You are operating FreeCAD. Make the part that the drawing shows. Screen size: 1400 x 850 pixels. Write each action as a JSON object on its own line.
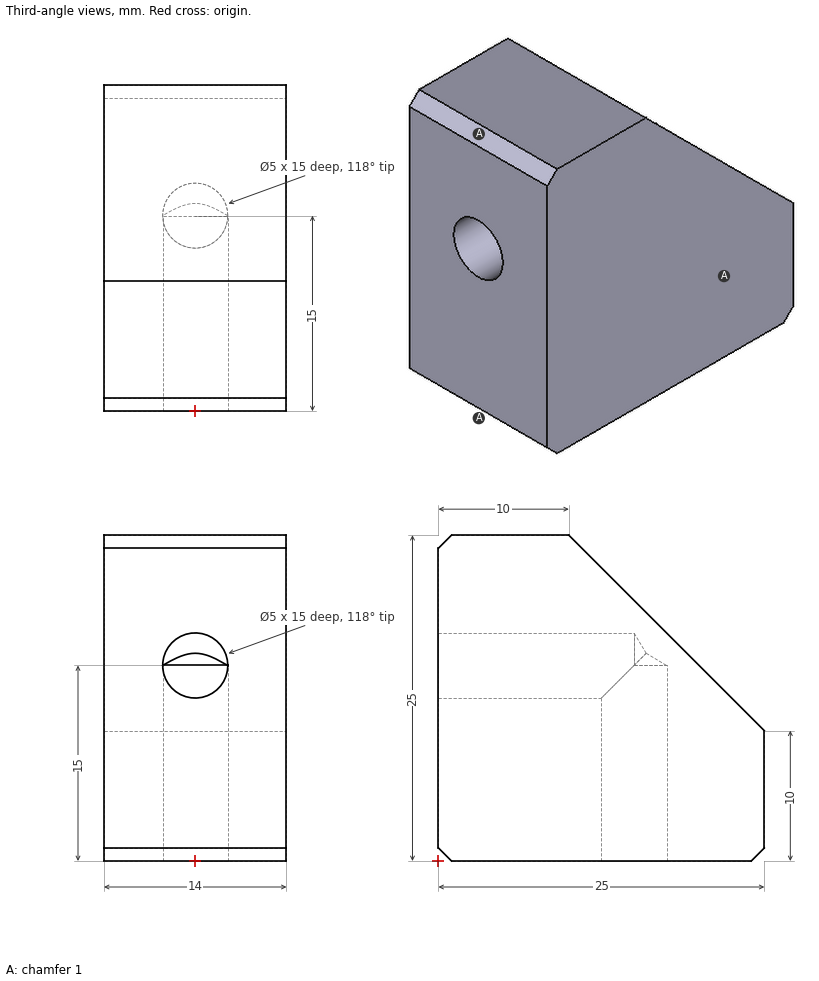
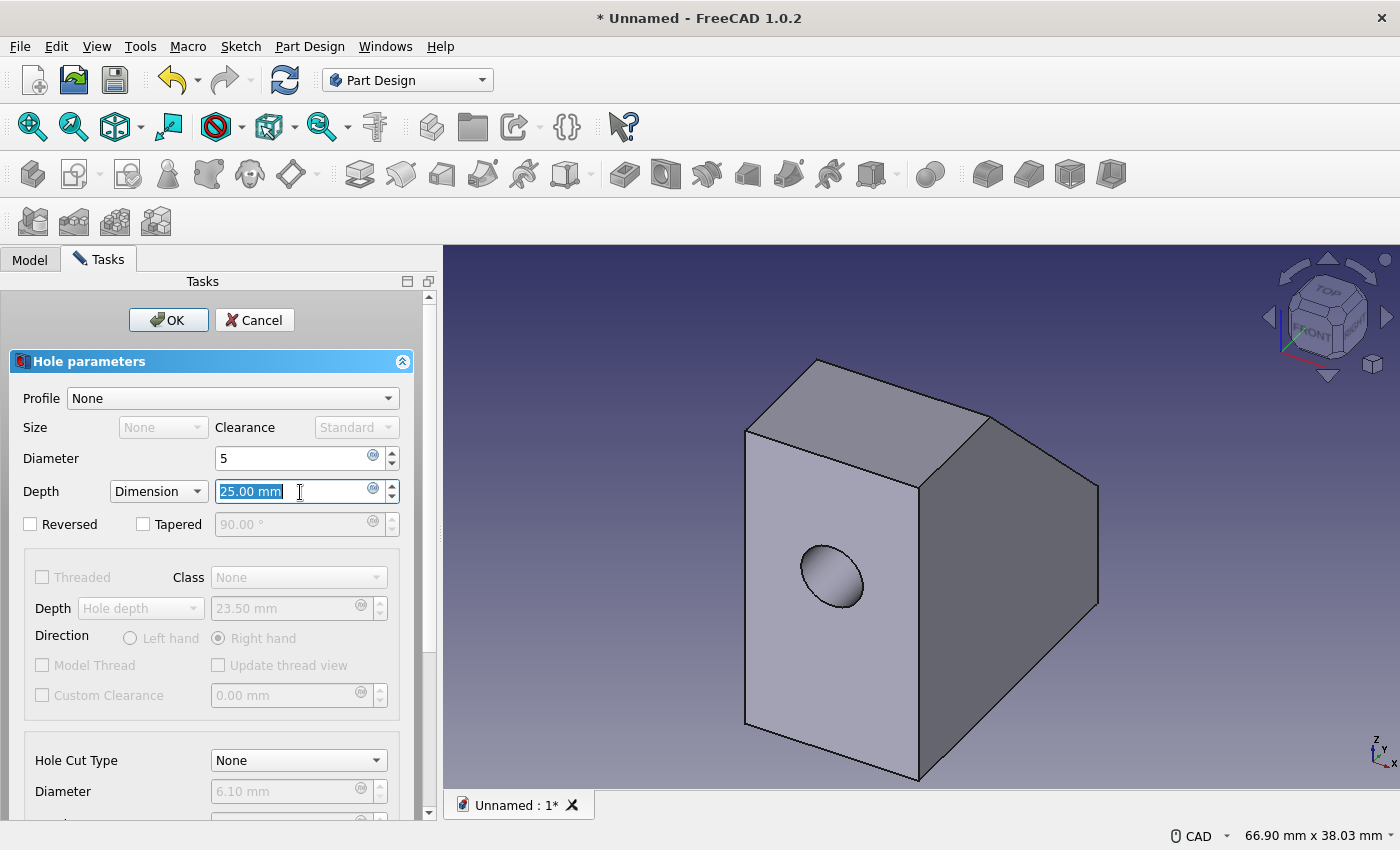
{"action": "type", "text": "15"}
{"action": "key", "text": "Tab"}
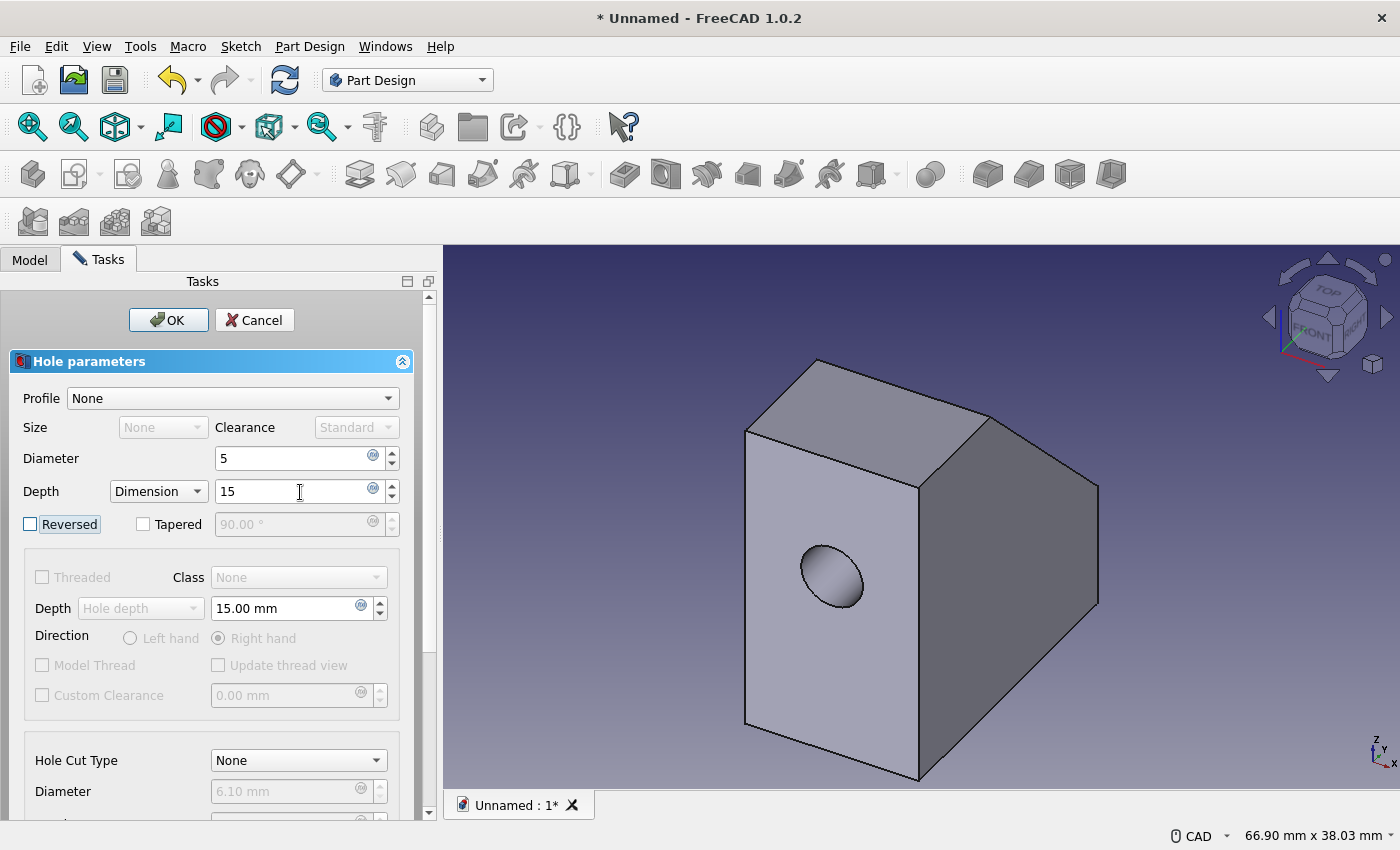
{"action": "left_click", "coordinate": [31, 524]}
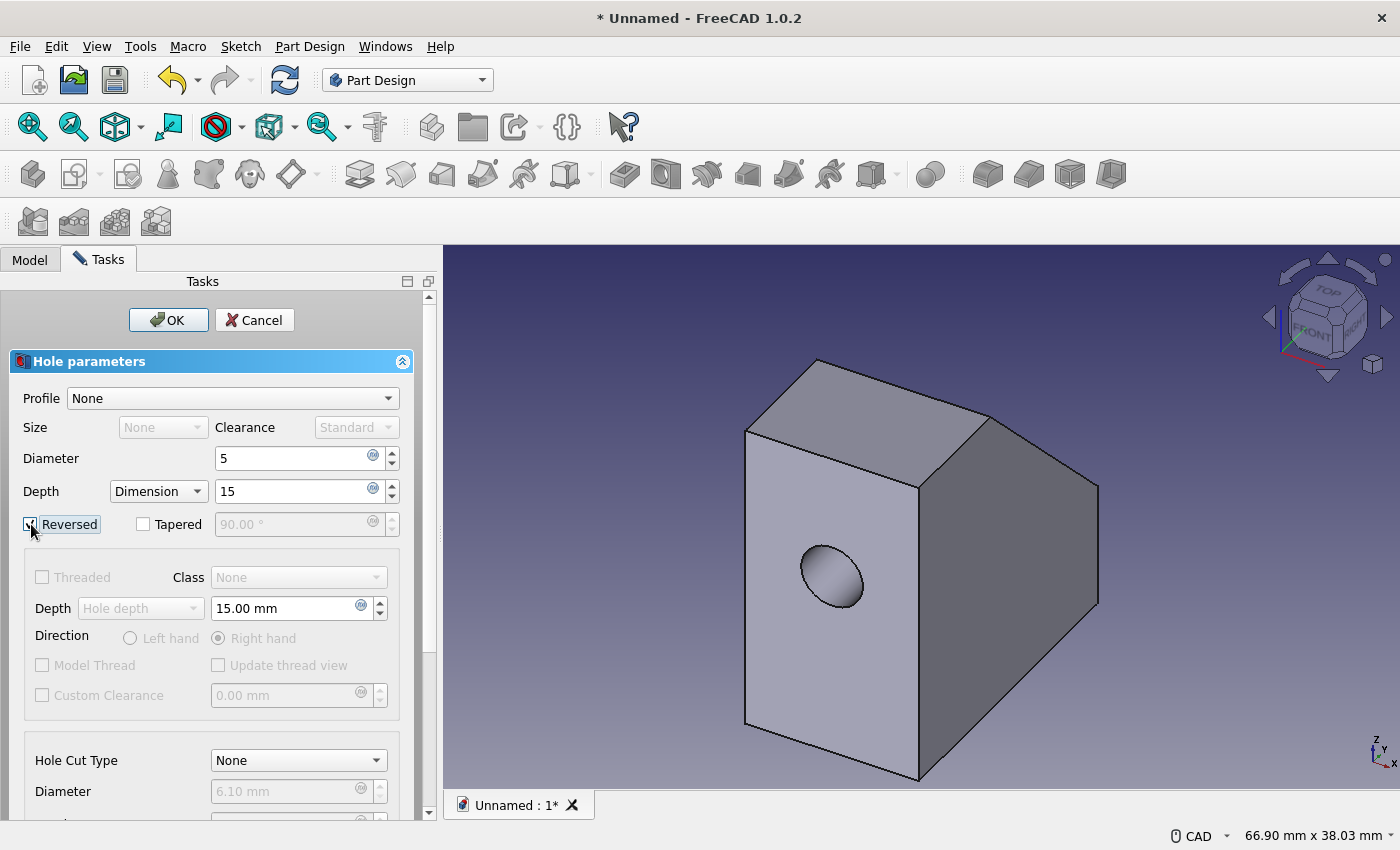
{"action": "left_click", "coordinate": [169, 320]}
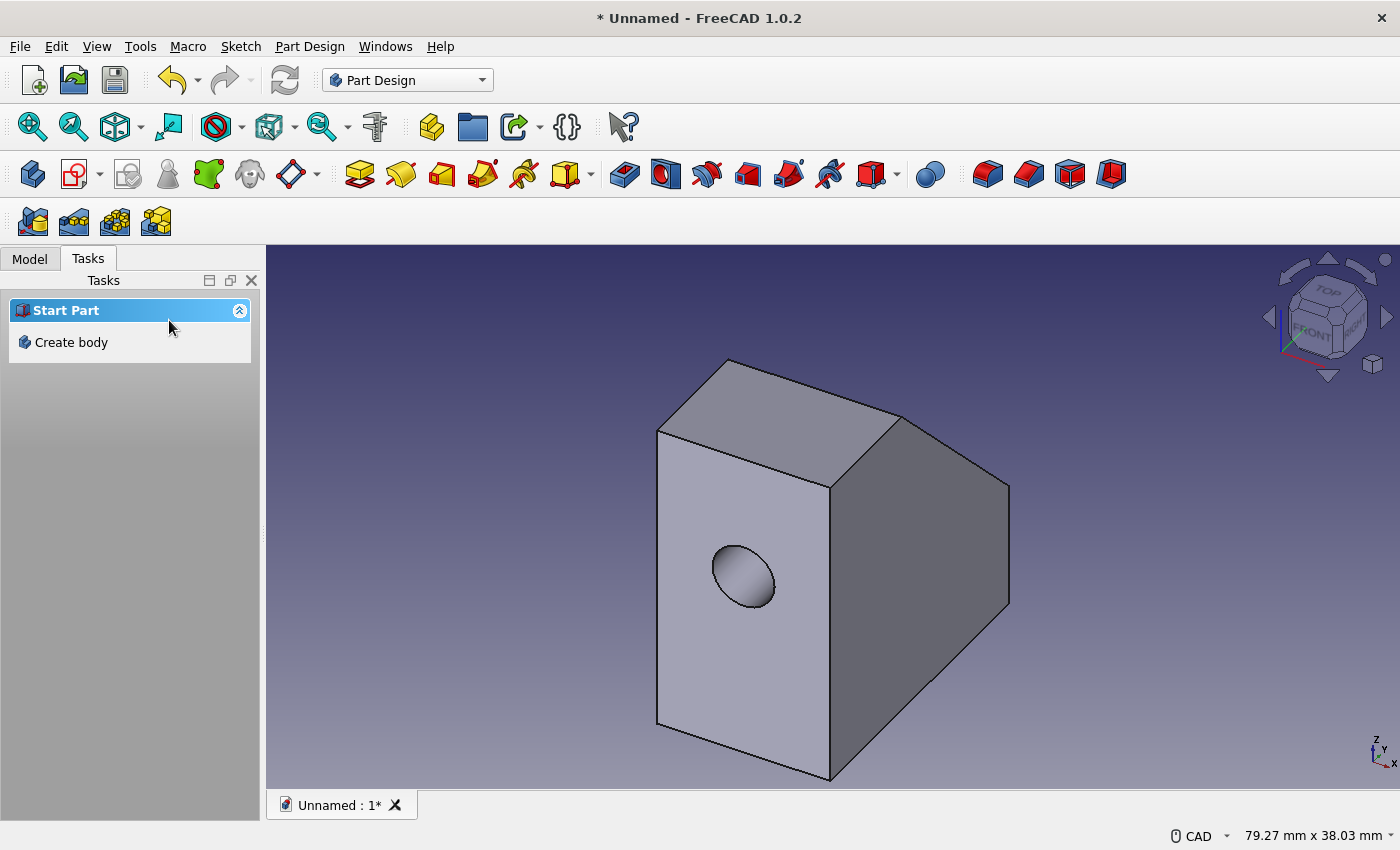
{"action": "left_click", "coordinate": [744, 458]}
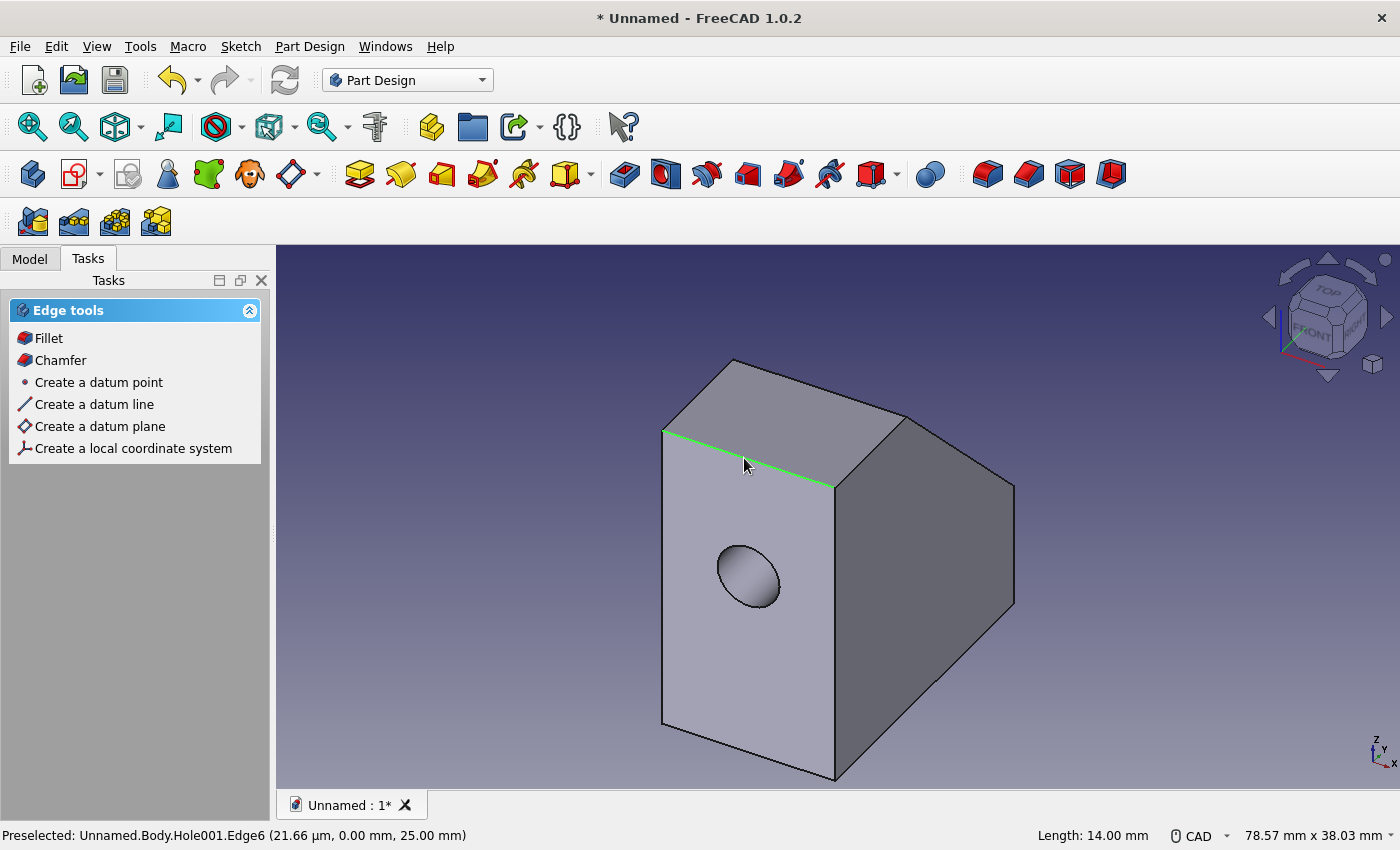
{"action": "key", "text": "0"}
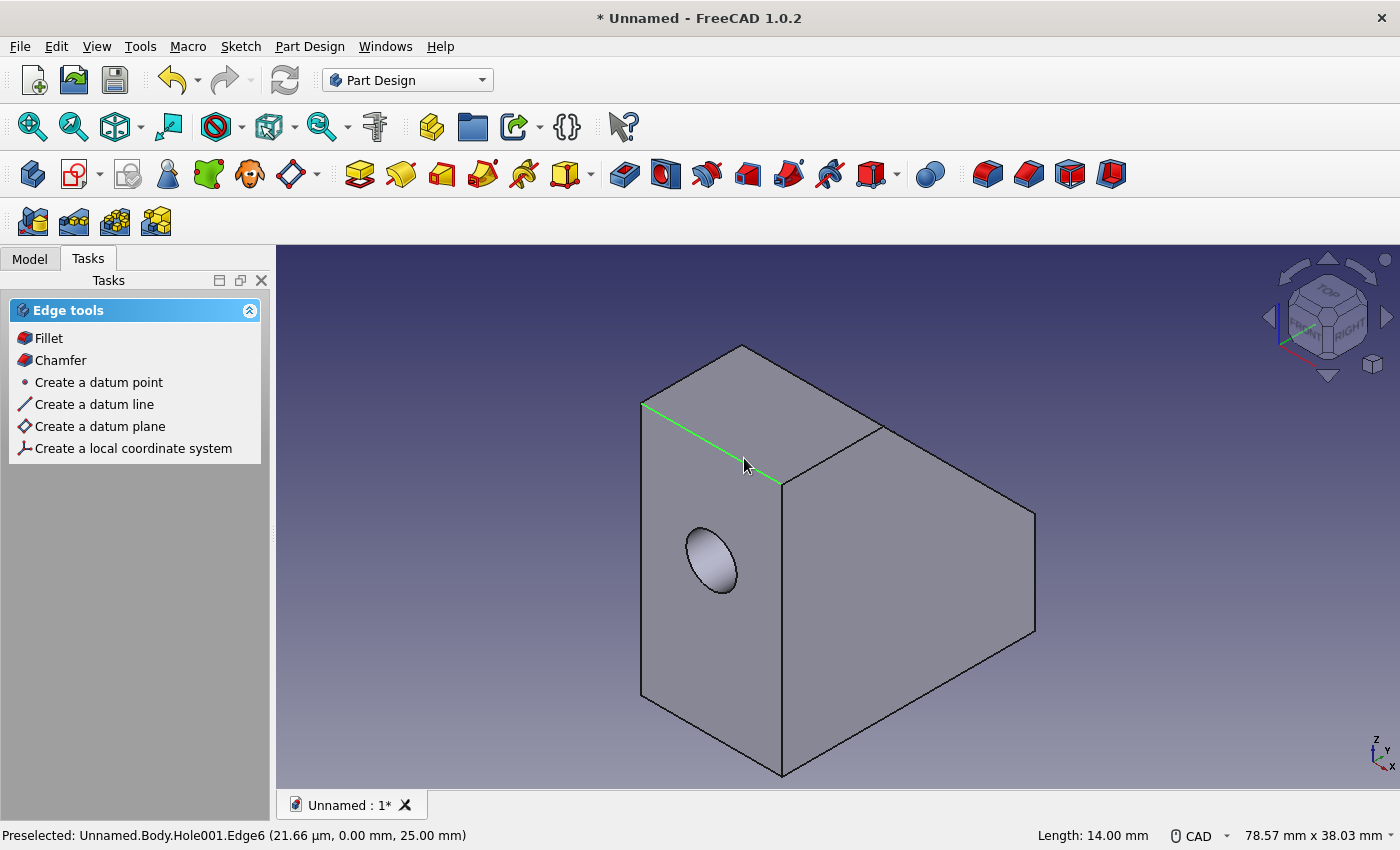
{"action": "key", "text": "2"}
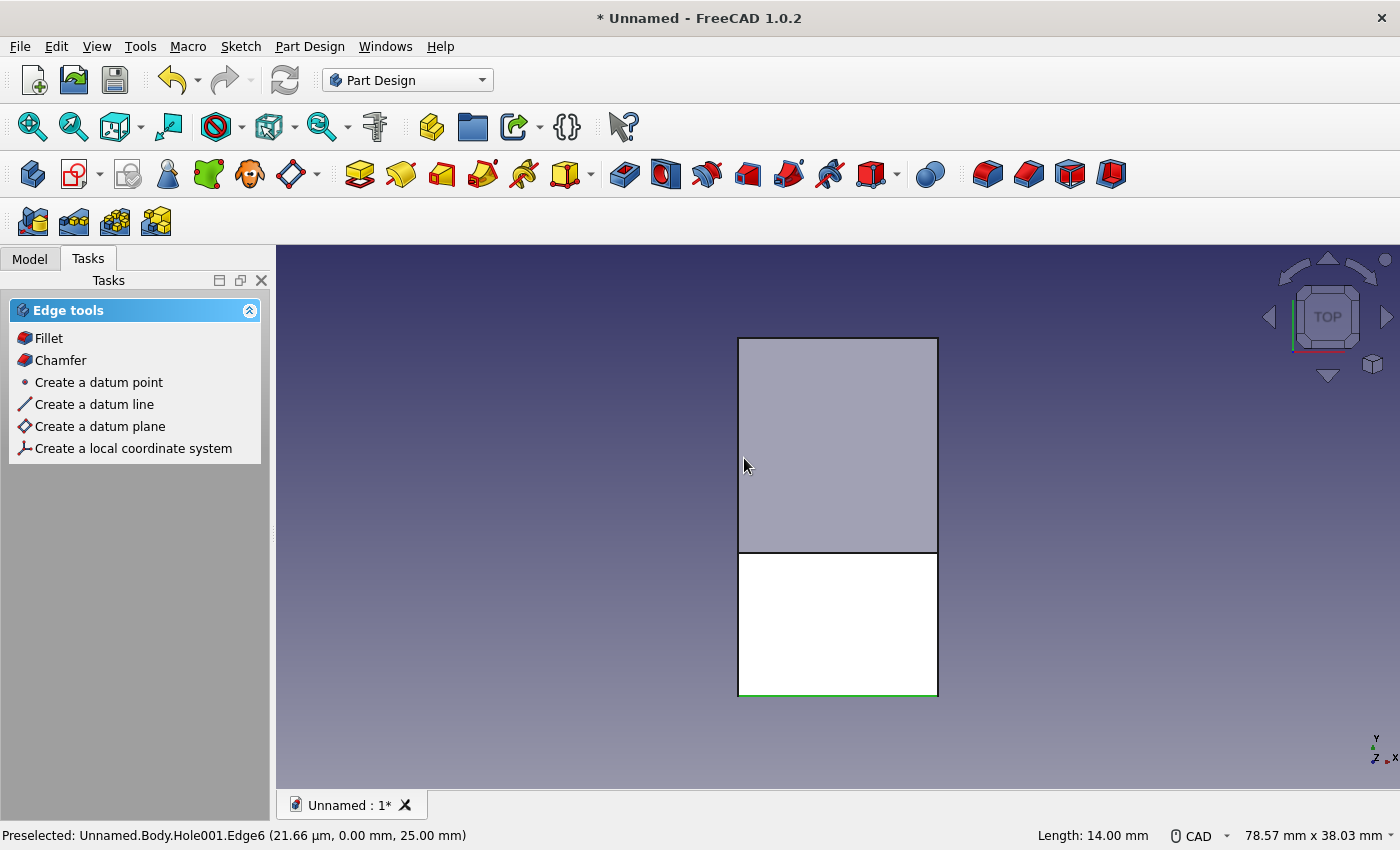
{"action": "key", "text": "1"}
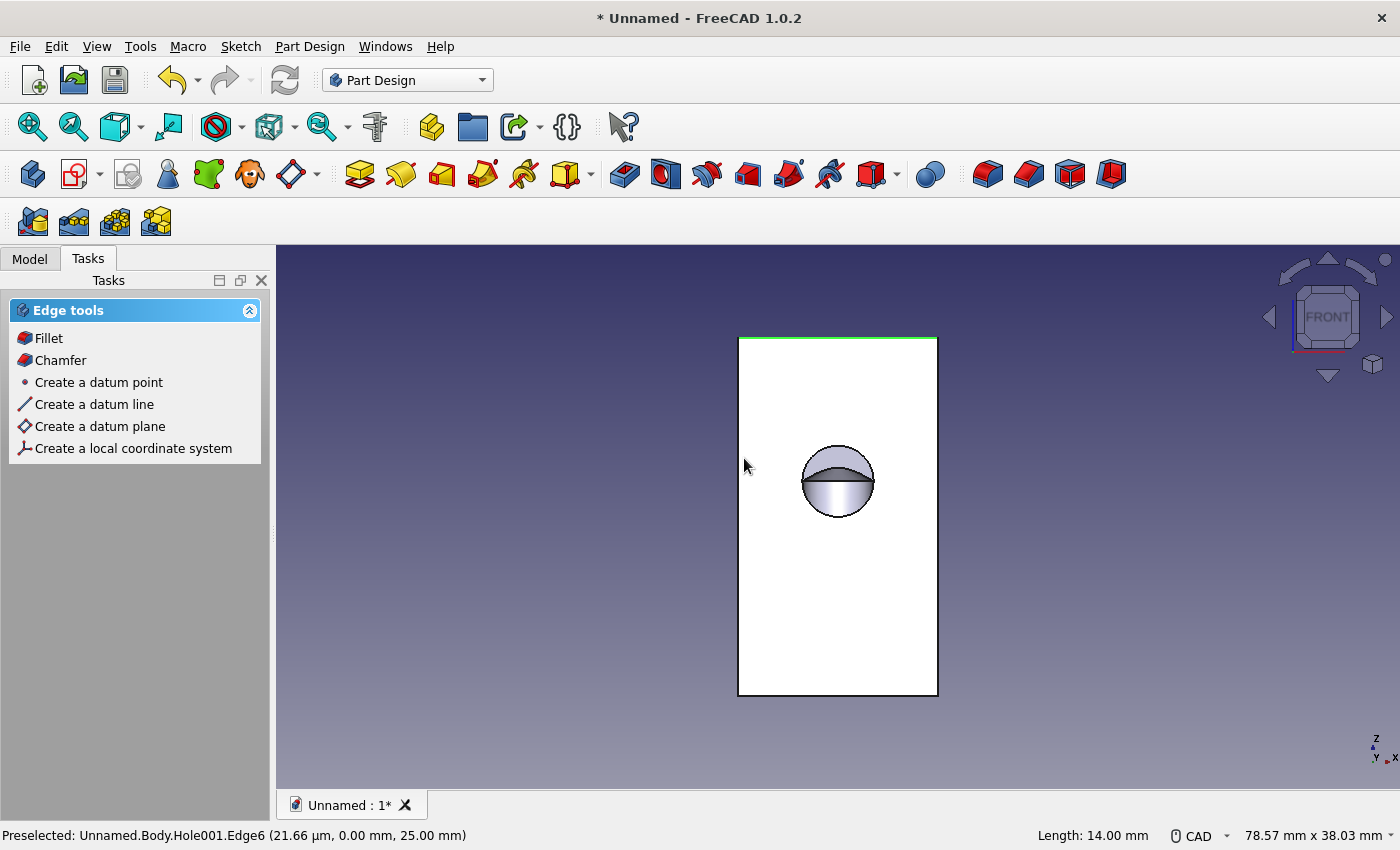
{"action": "left_click", "coordinate": [838, 695], "text": "ctrl"}